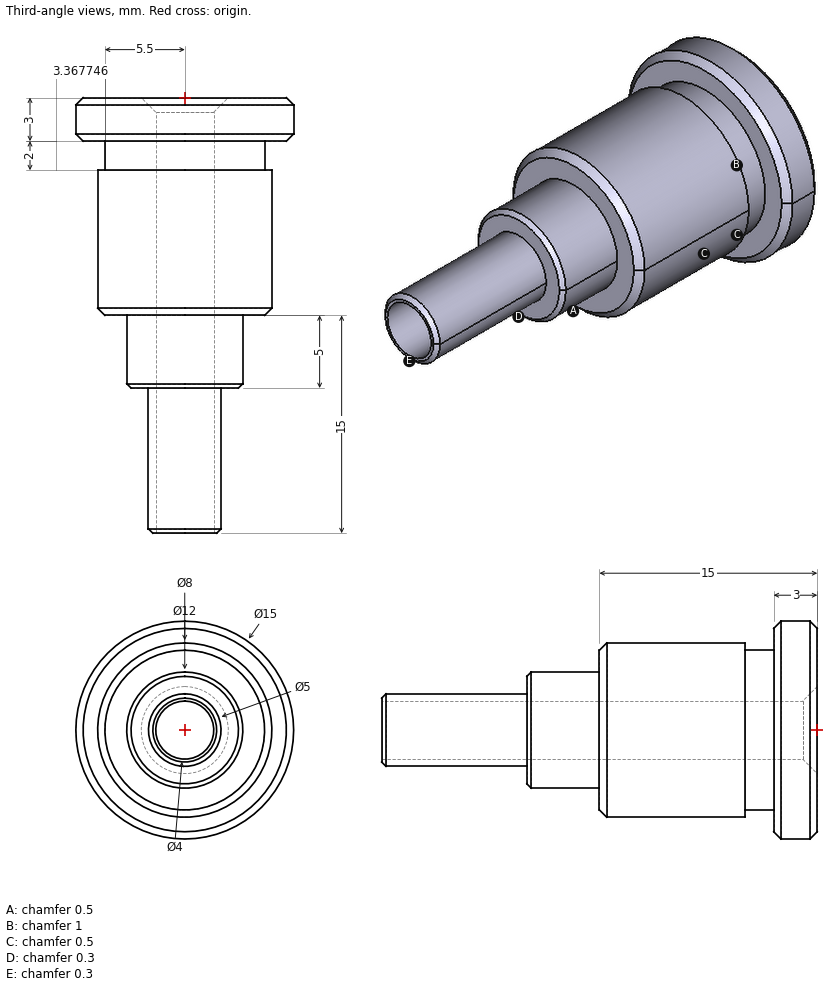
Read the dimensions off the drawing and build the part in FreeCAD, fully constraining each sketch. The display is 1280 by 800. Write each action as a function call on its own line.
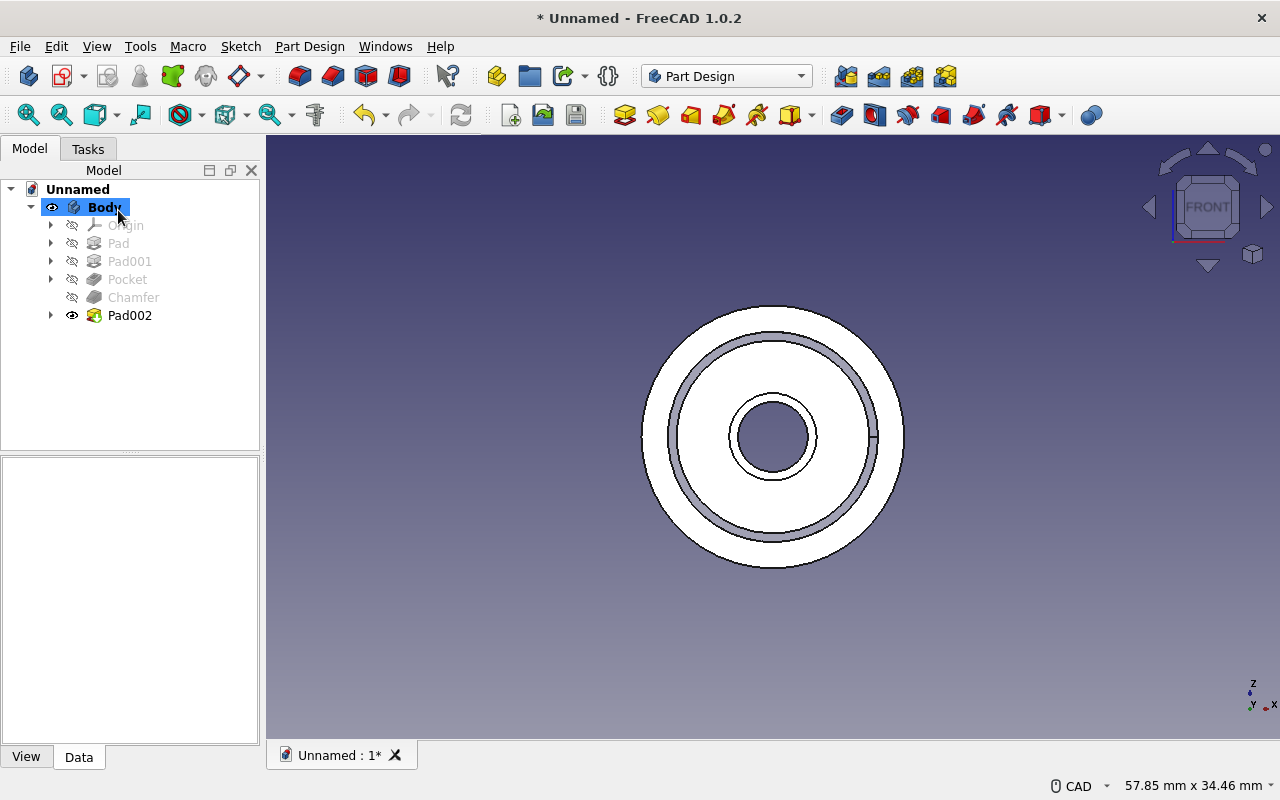
click(29, 116)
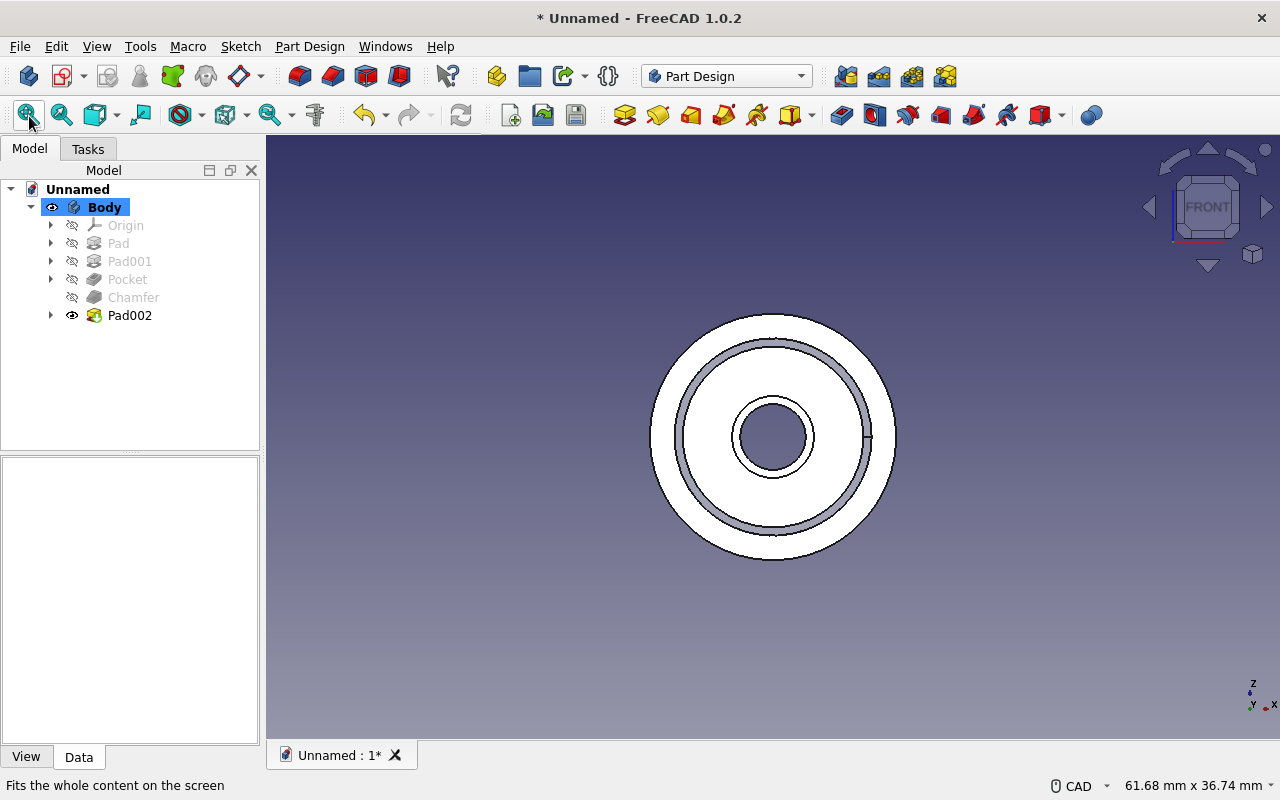
key(3)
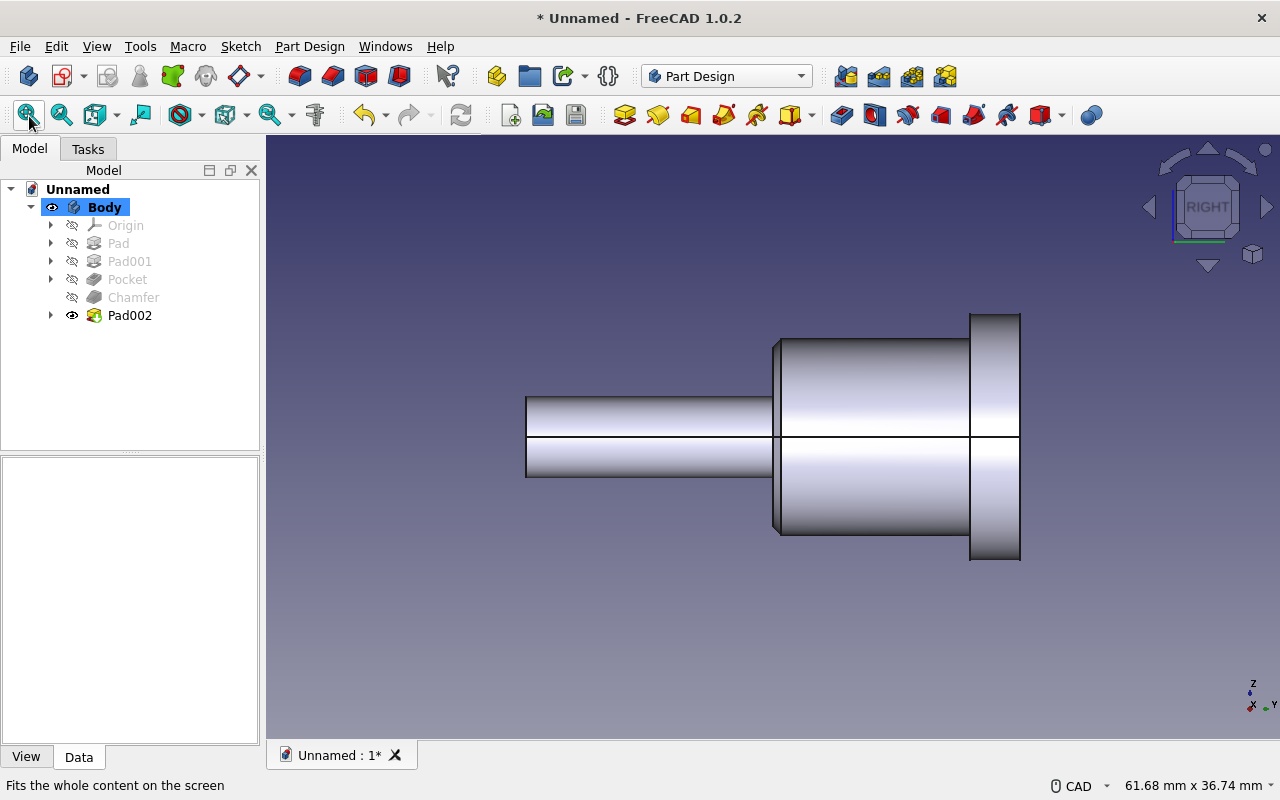
key(5)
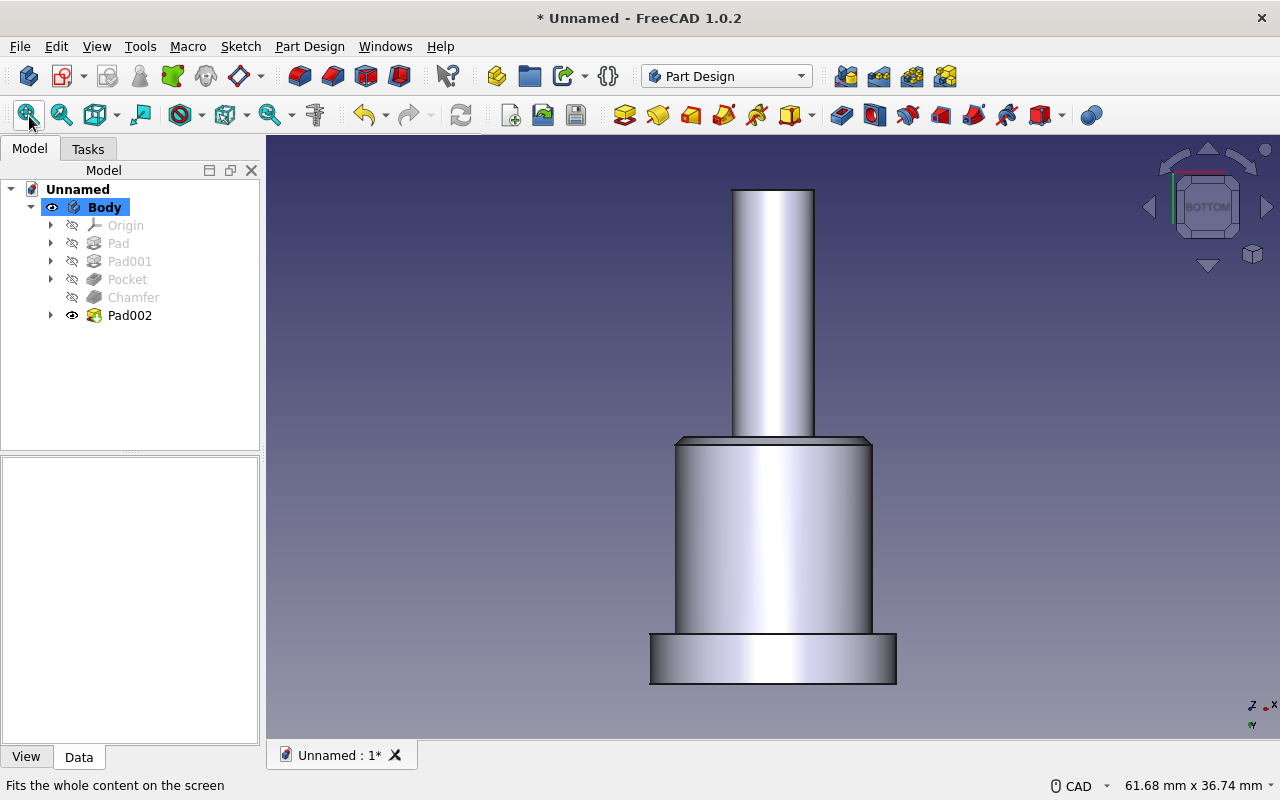
key(4)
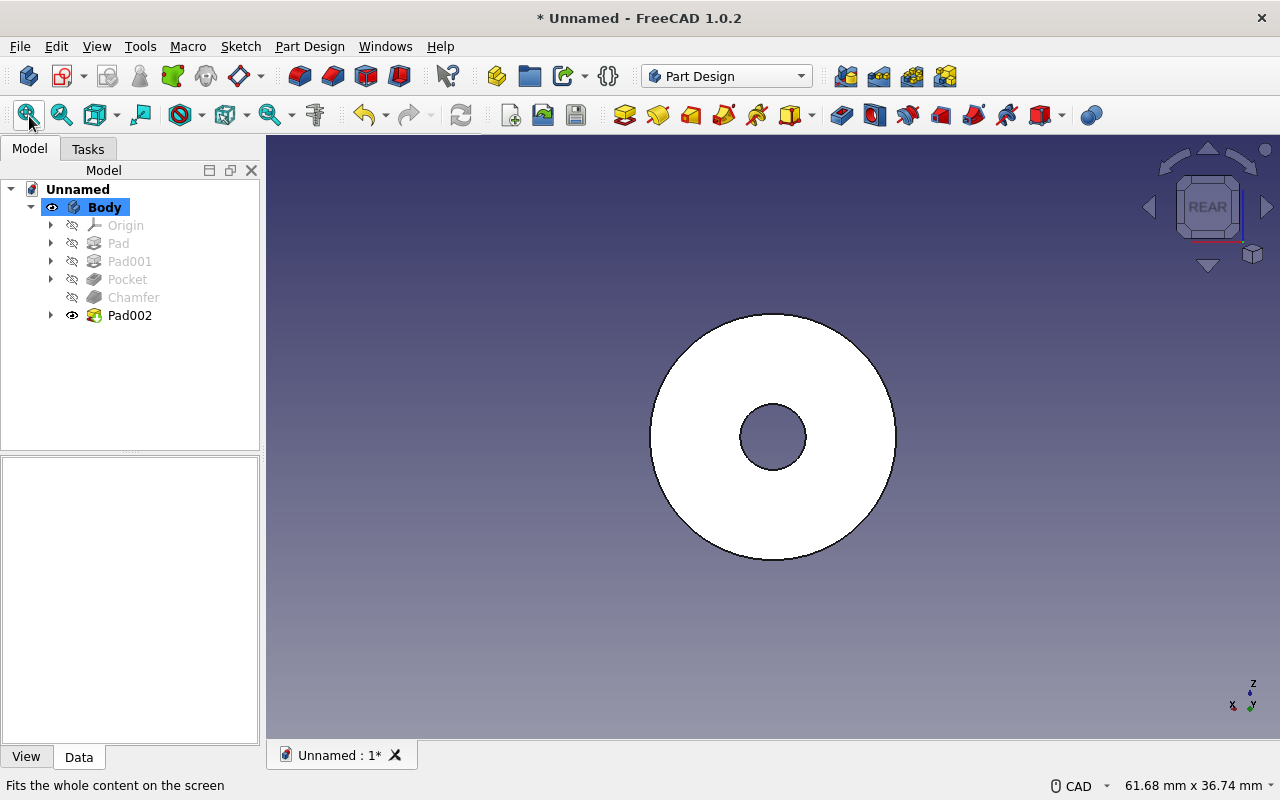
click(29, 116)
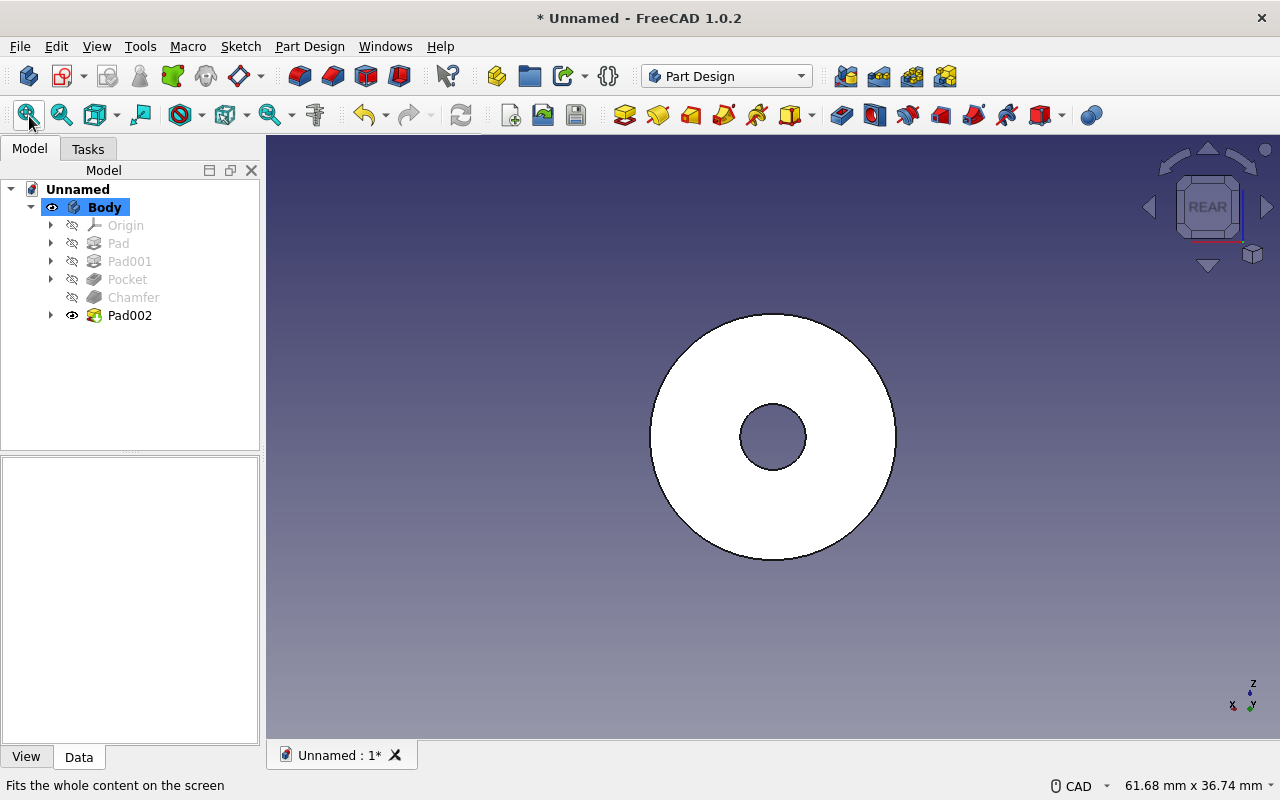
click(800, 417)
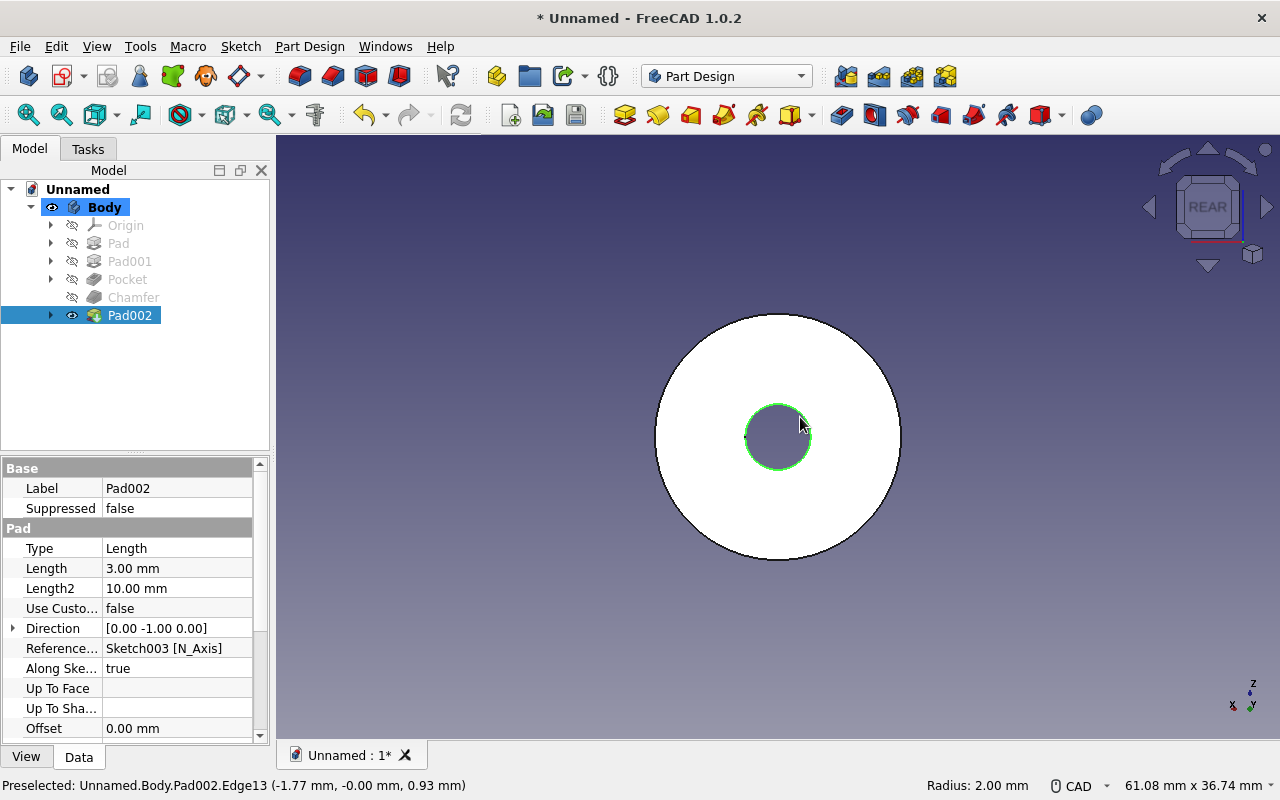
click(333, 76)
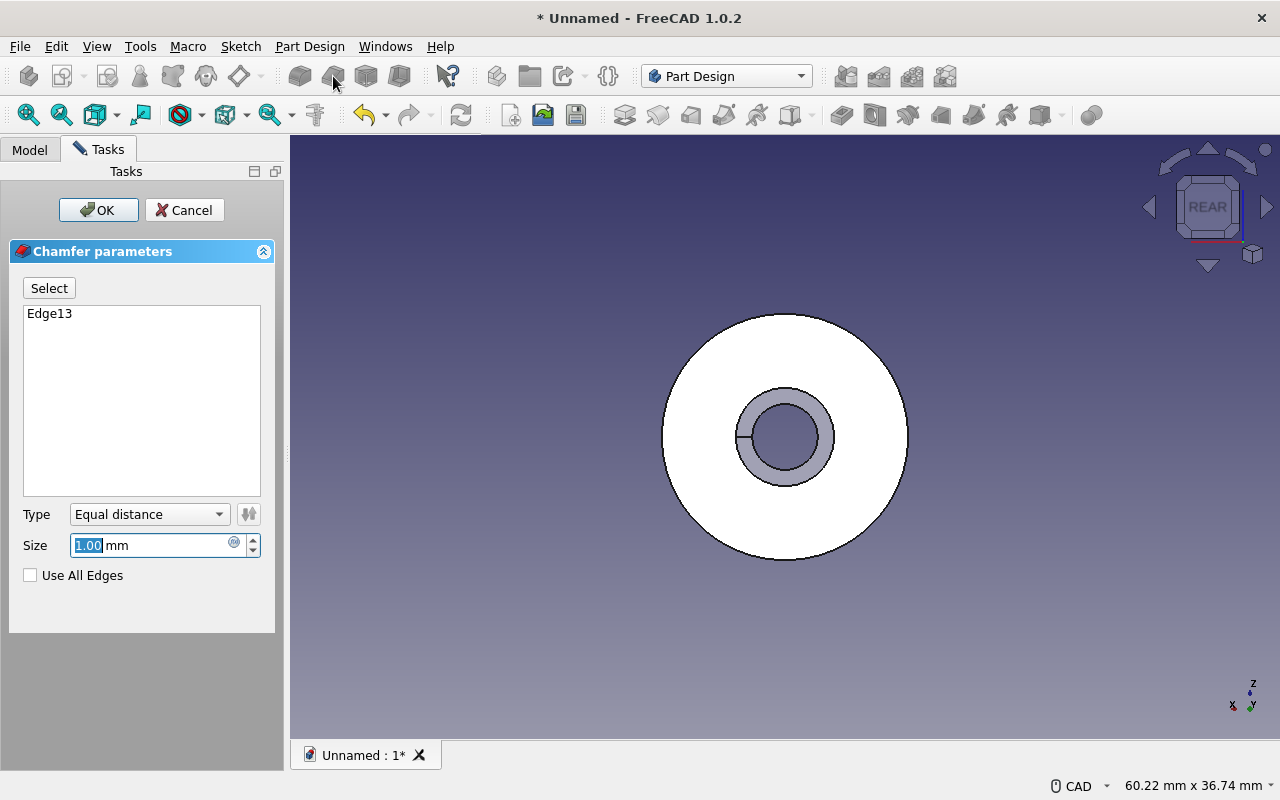
text(1)
key(Tab)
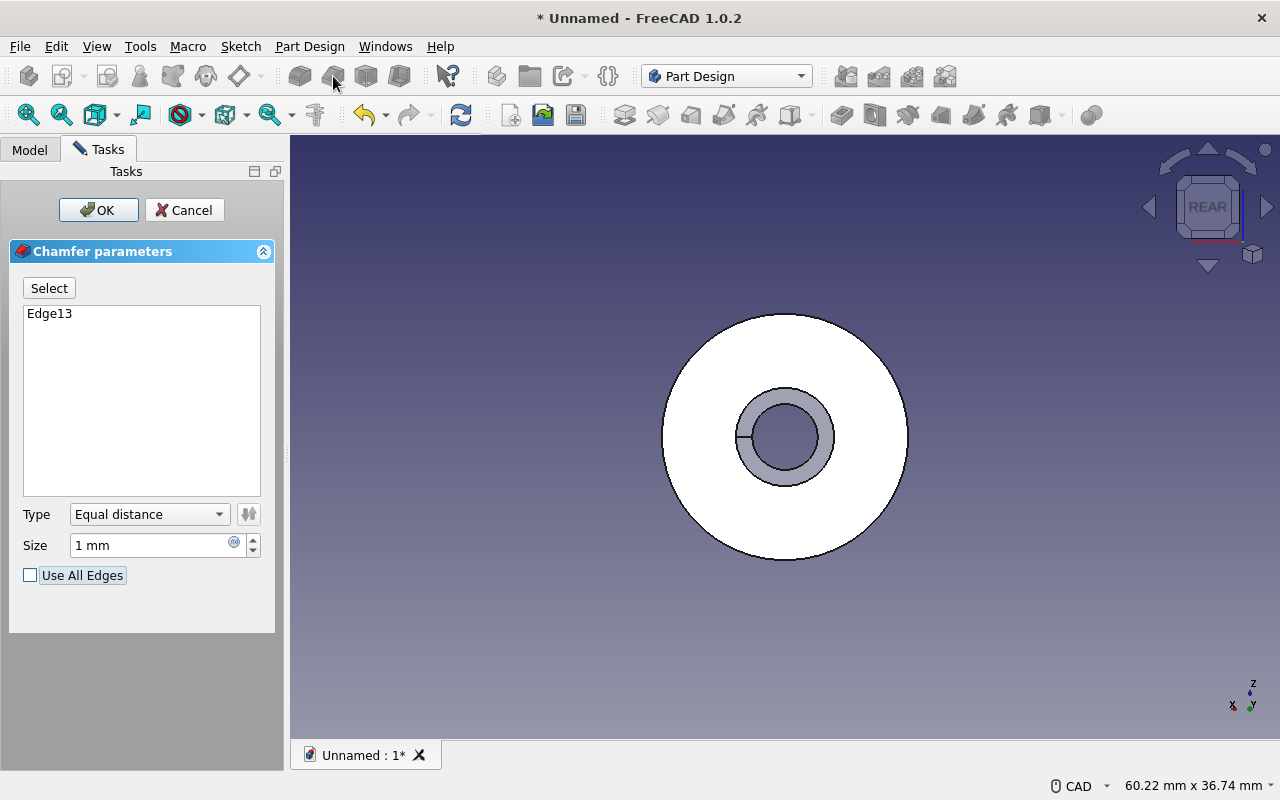
click(99, 210)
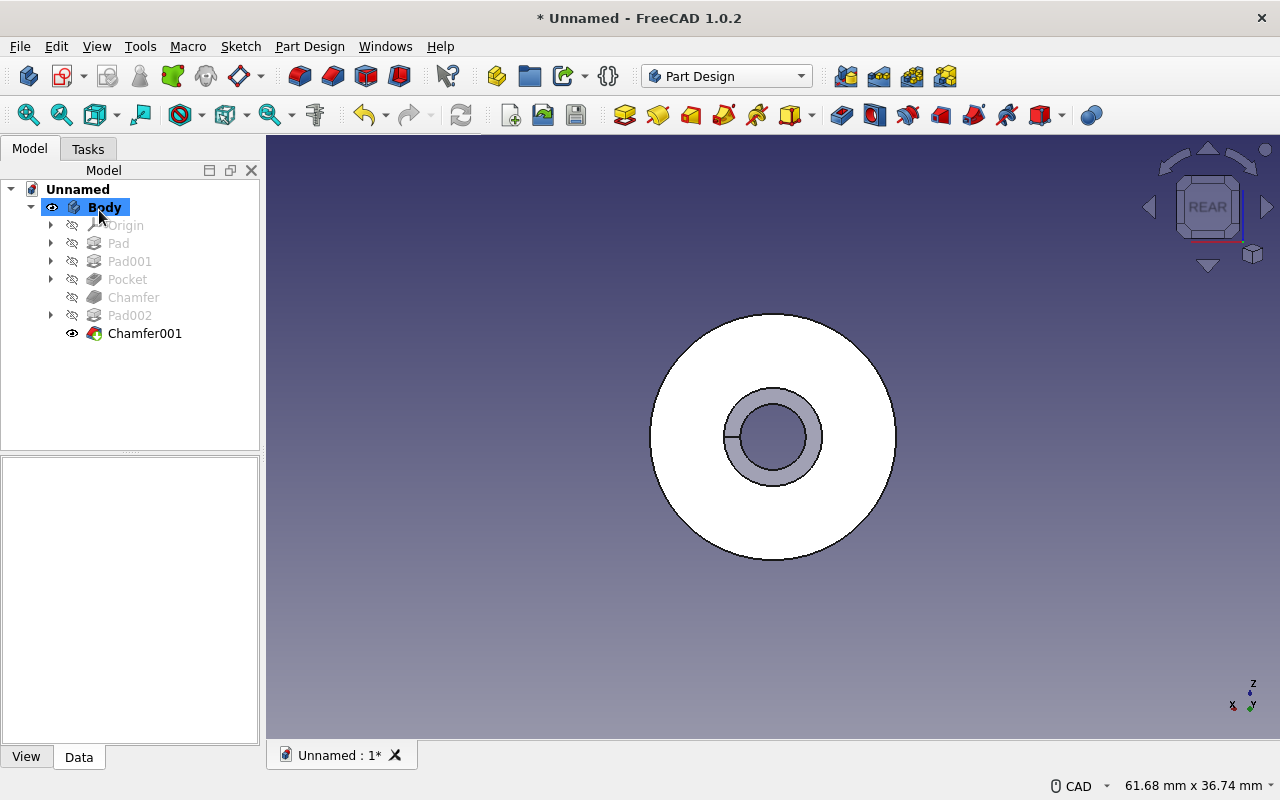
click(29, 116)